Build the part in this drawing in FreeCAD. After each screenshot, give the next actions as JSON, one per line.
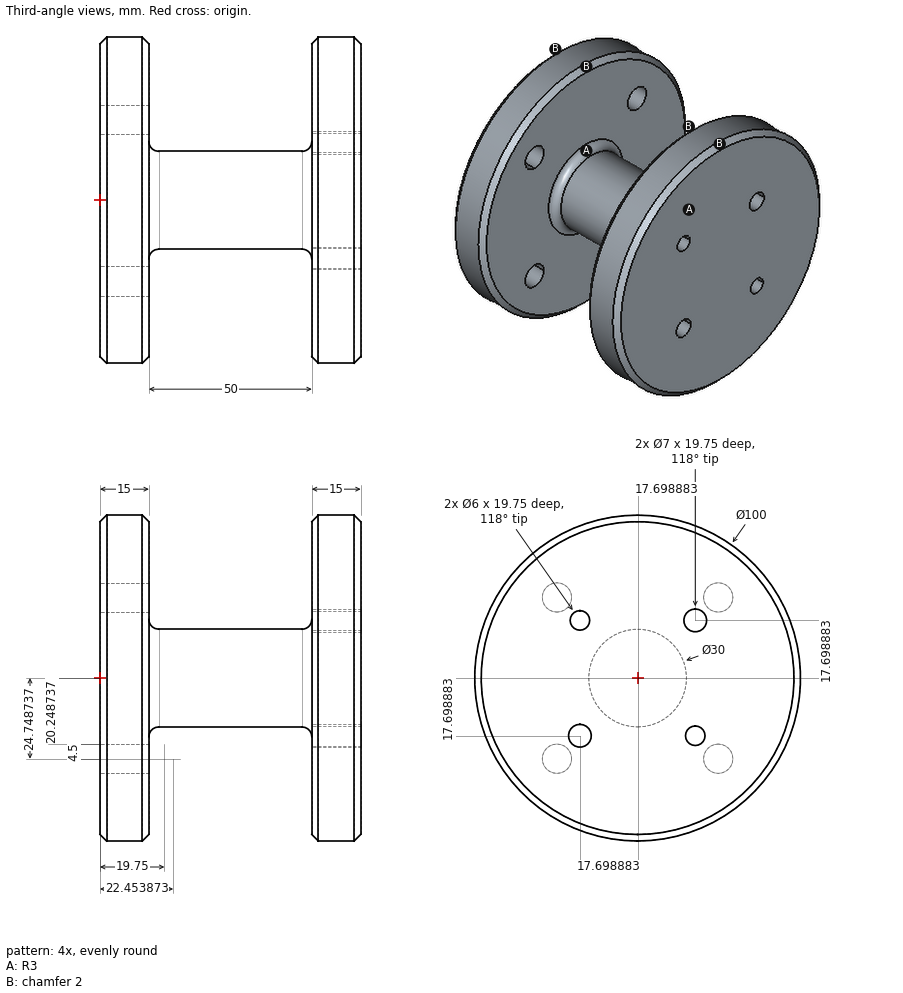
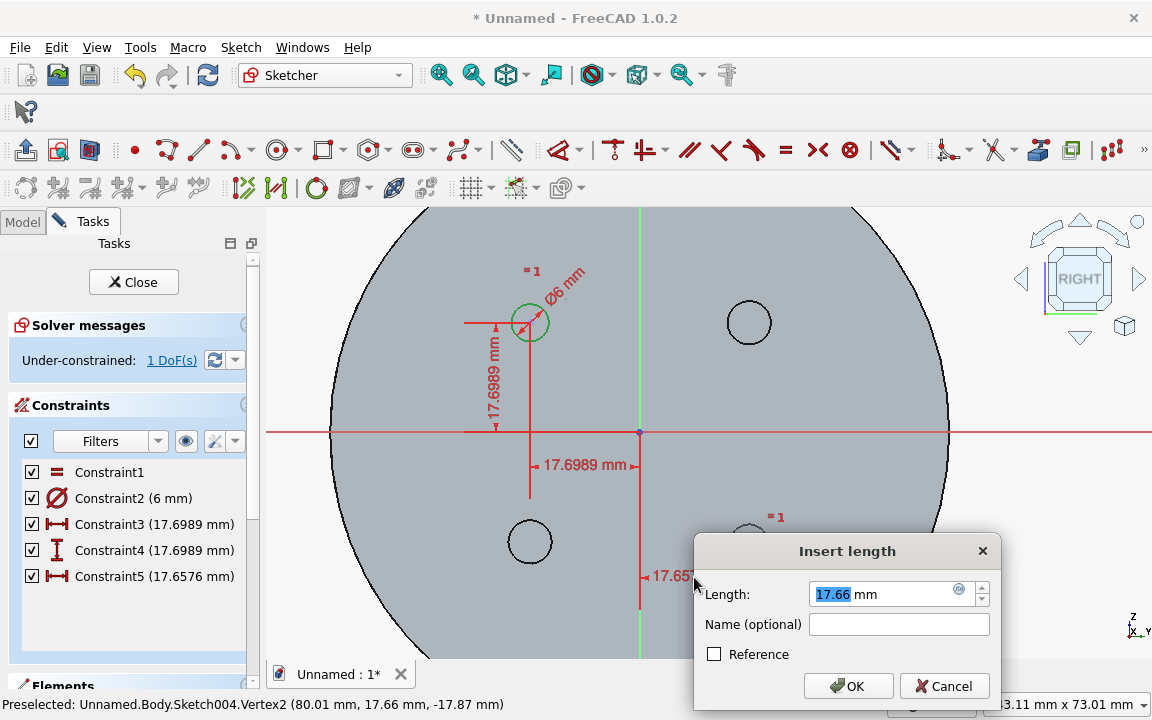
{"action": "type", "text": "17.698883"}
{"action": "key", "text": "Return"}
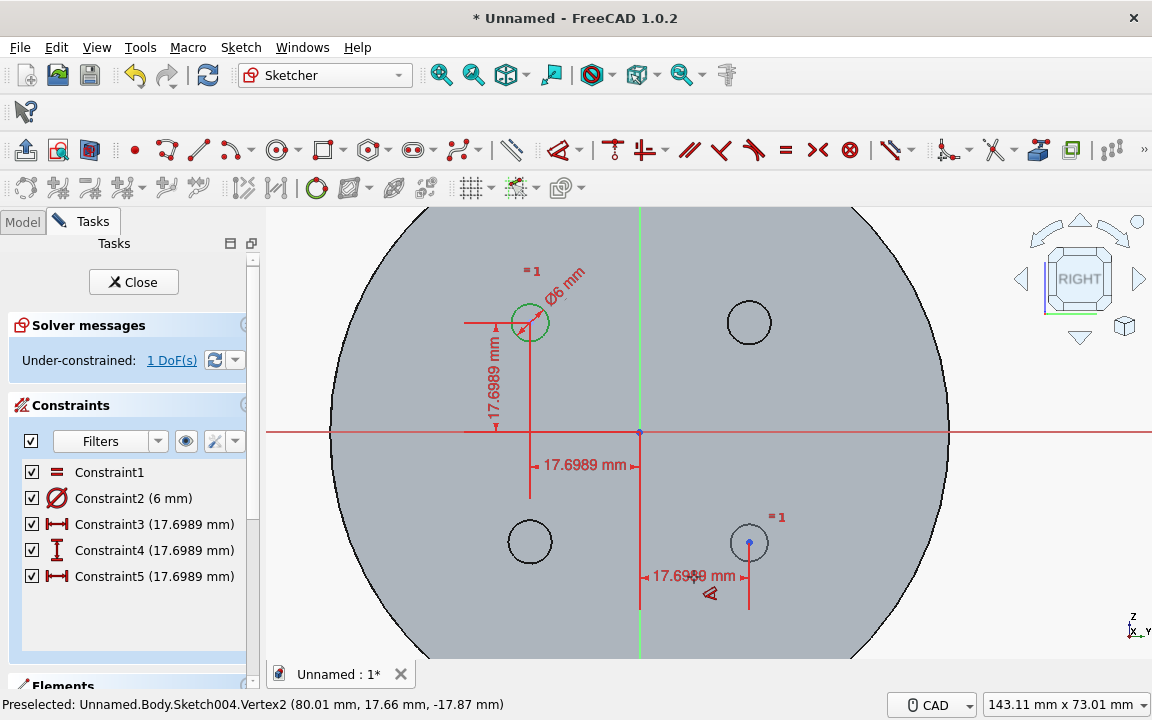
{"action": "left_click", "coordinate": [749, 543]}
{"action": "left_click", "coordinate": [783, 488]}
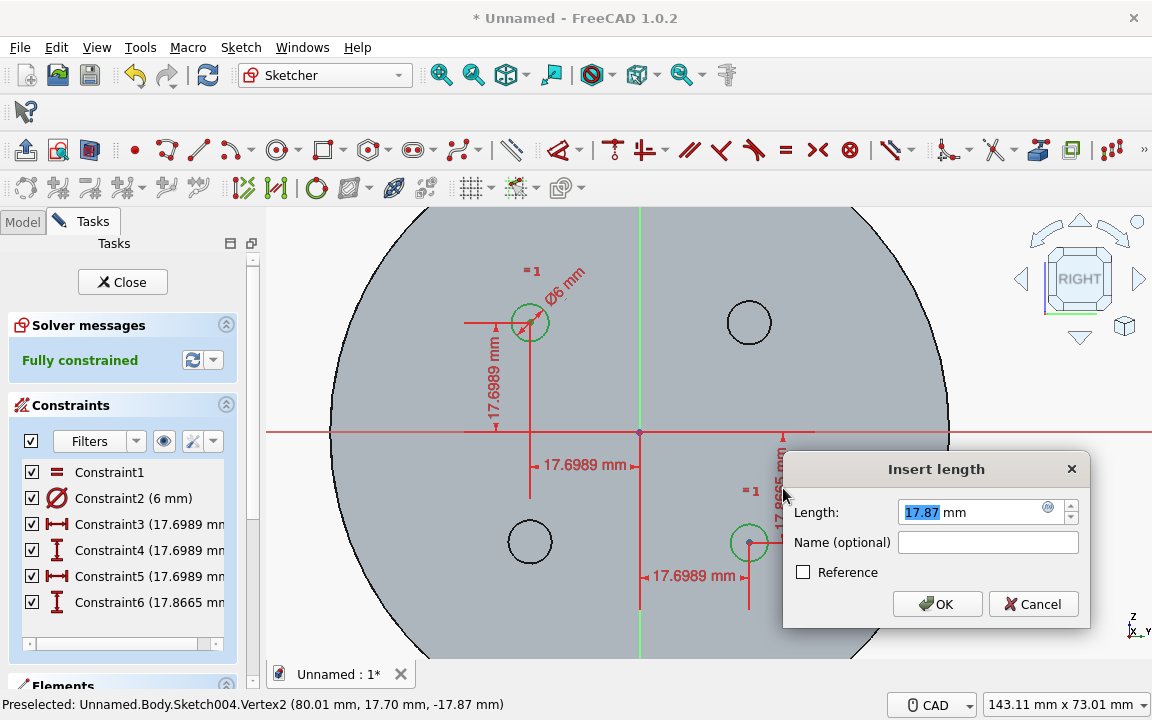
{"action": "type", "text": "17.698883"}
{"action": "key", "text": "Return"}
{"action": "key", "text": "Escape"}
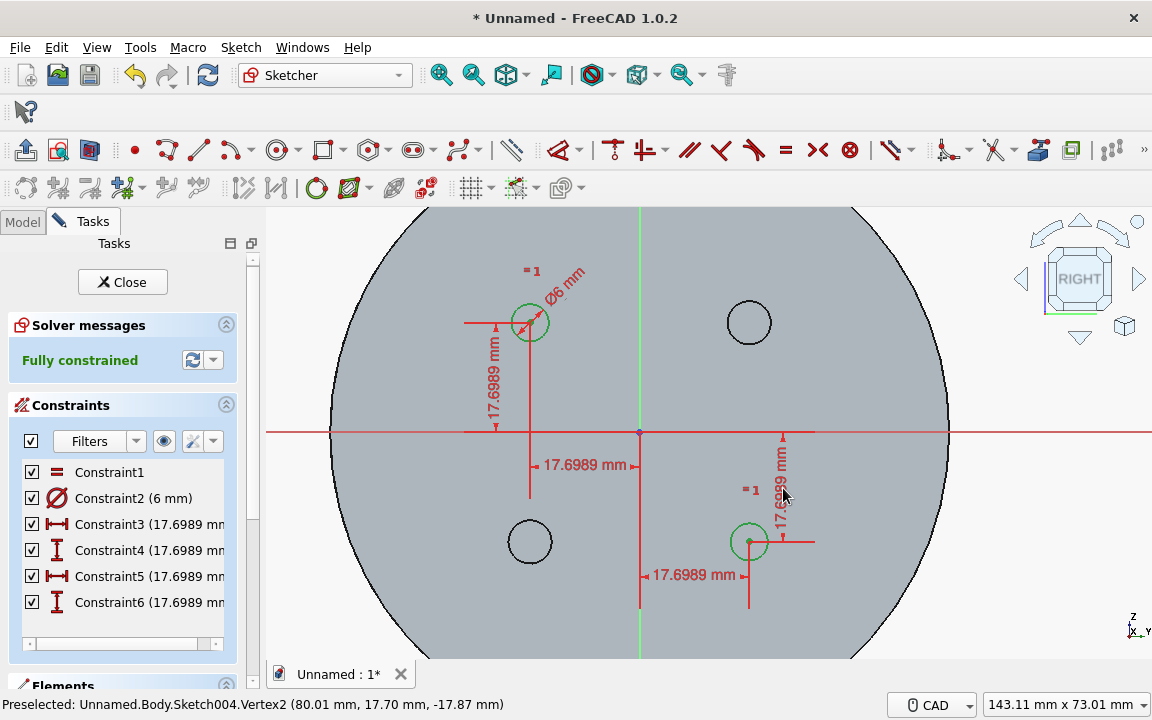
{"action": "left_click", "coordinate": [123, 282]}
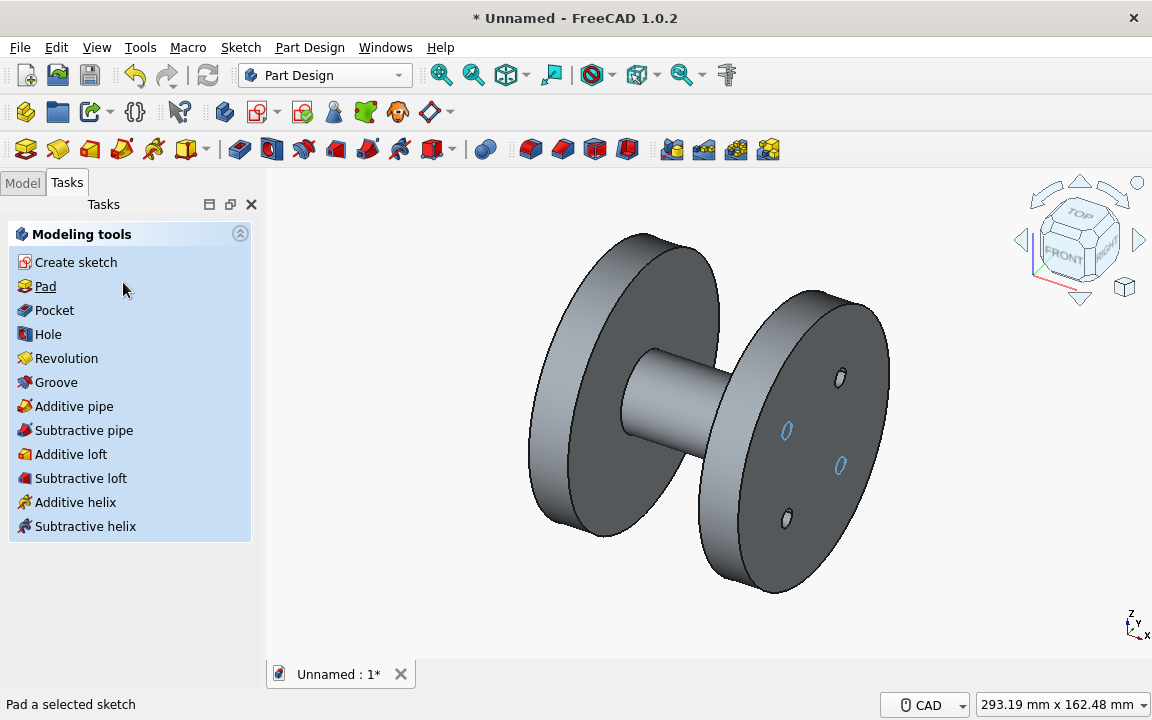
{"action": "left_click", "coordinate": [272, 150]}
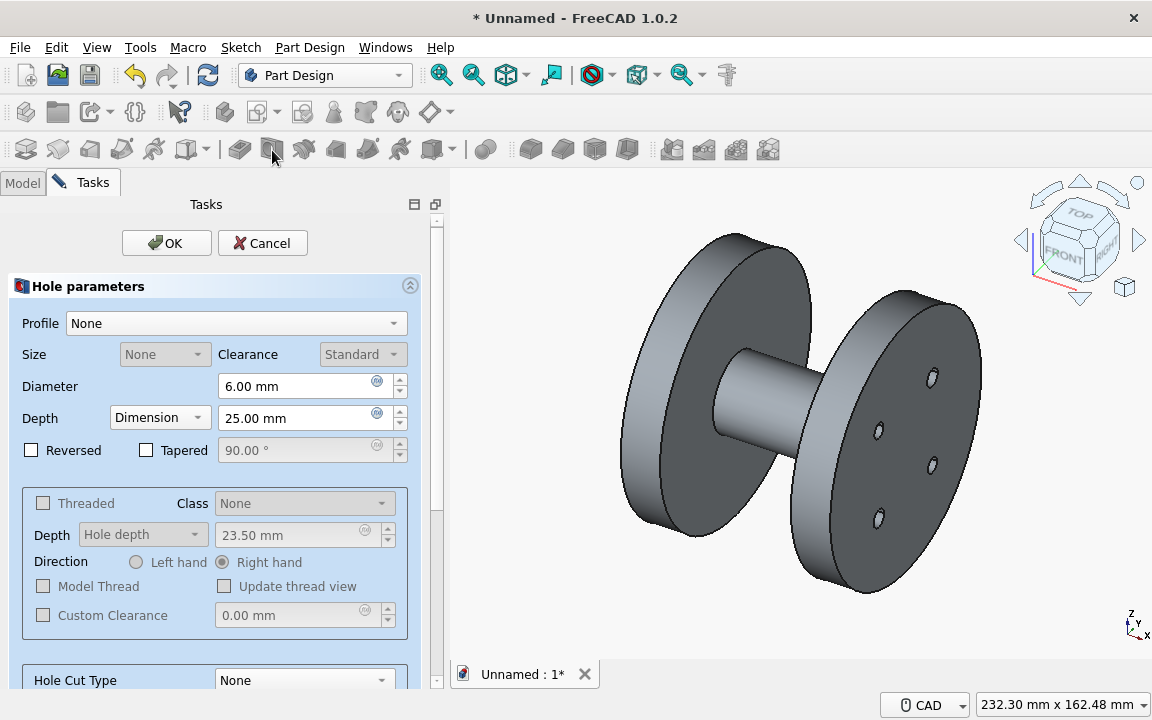
{"action": "triple_click", "coordinate": [305, 386]}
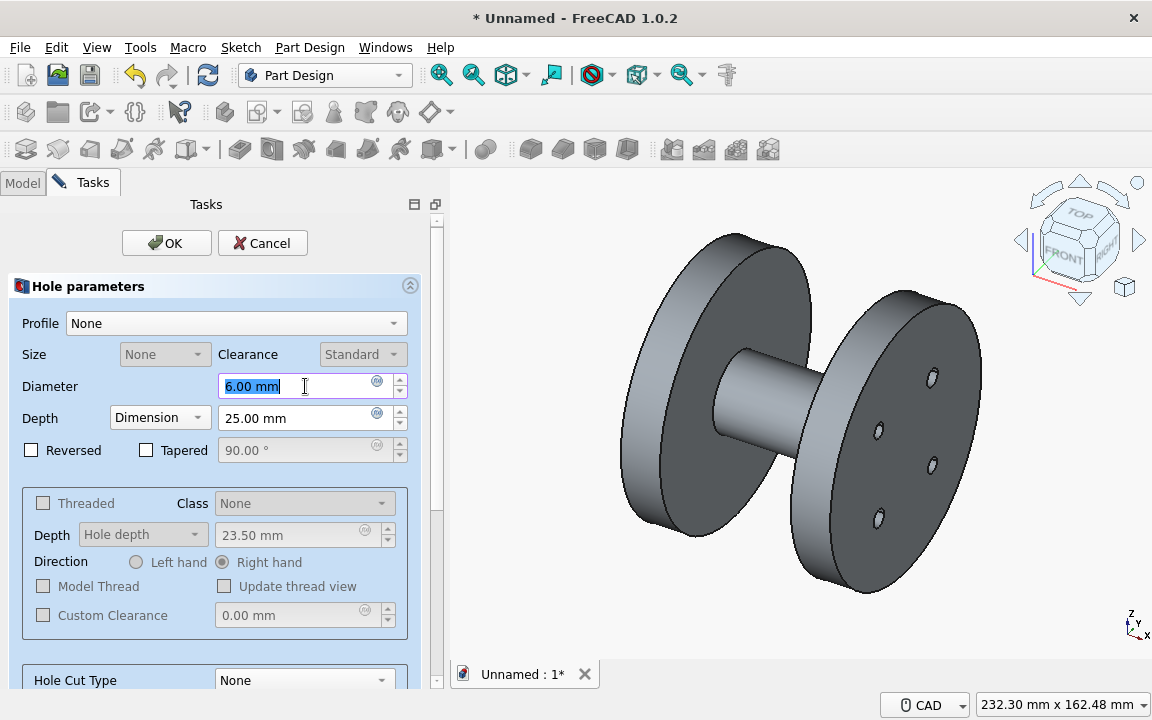
{"action": "type", "text": "6"}
{"action": "key", "text": "Tab"}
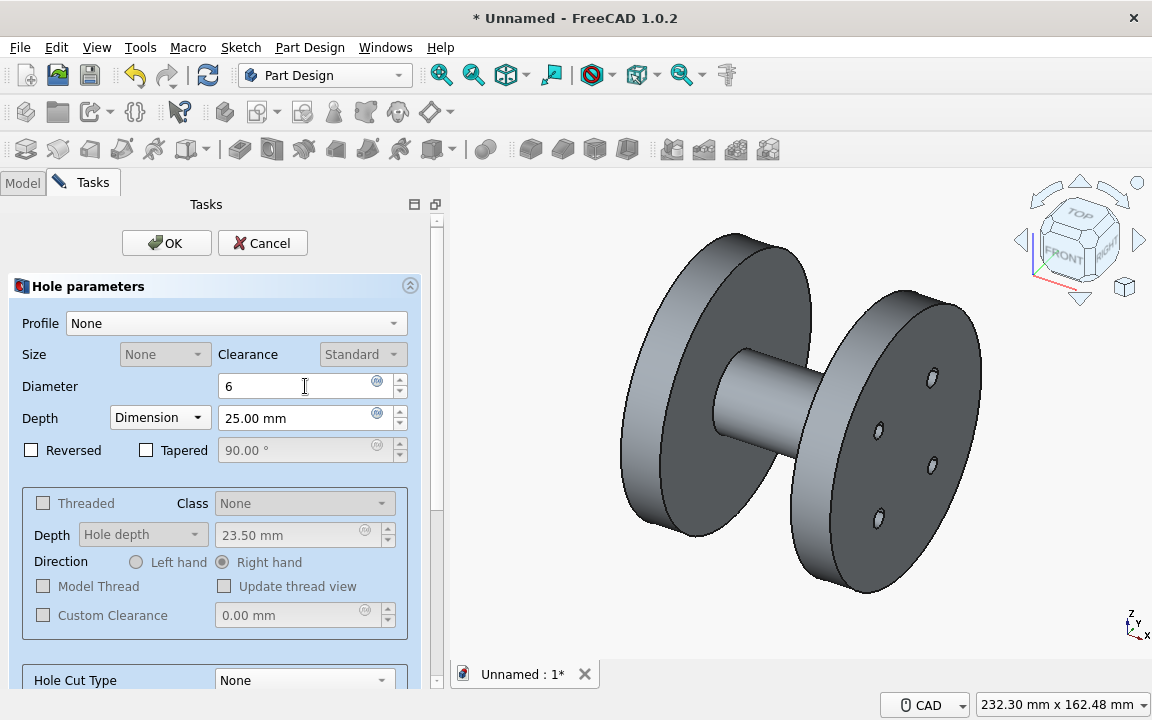
{"action": "triple_click", "coordinate": [305, 418]}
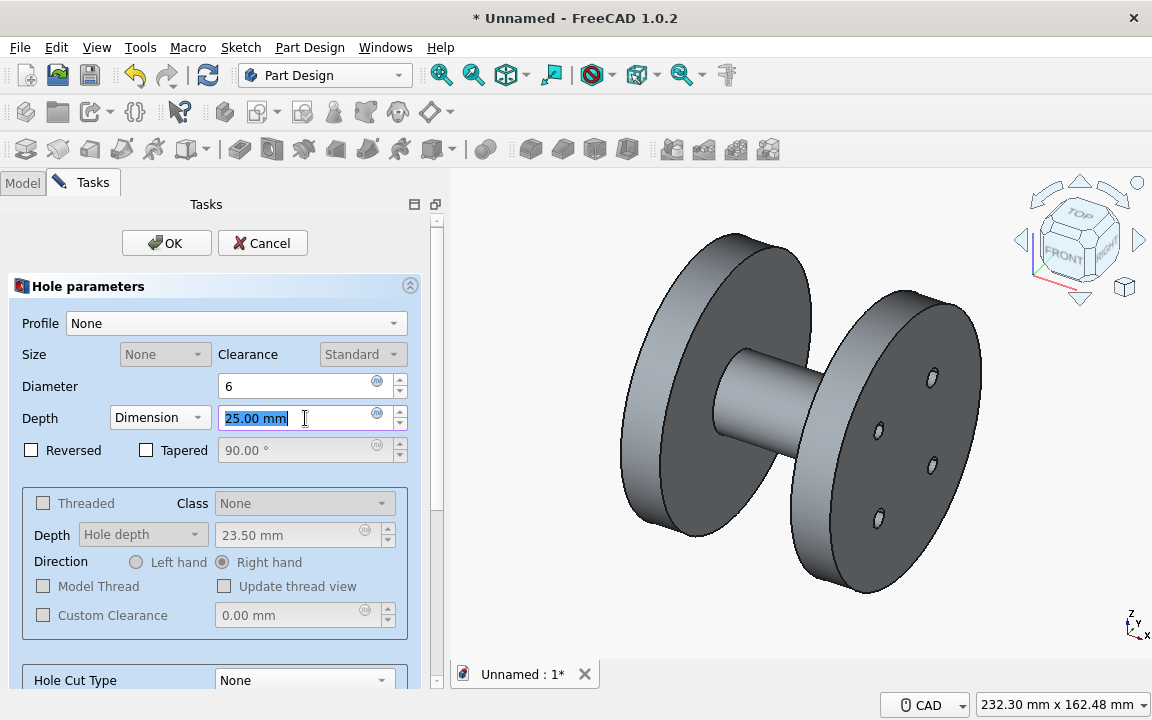
{"action": "type", "text": "19.75"}
{"action": "key", "text": "Tab"}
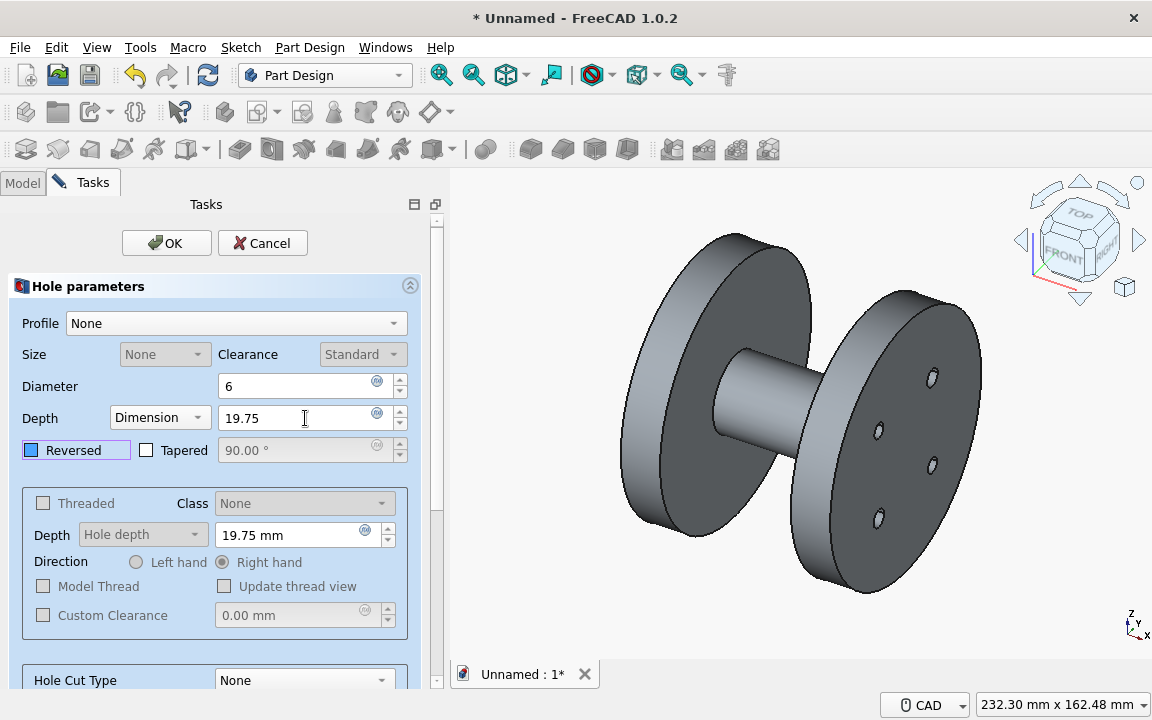
{"action": "left_click", "coordinate": [167, 243]}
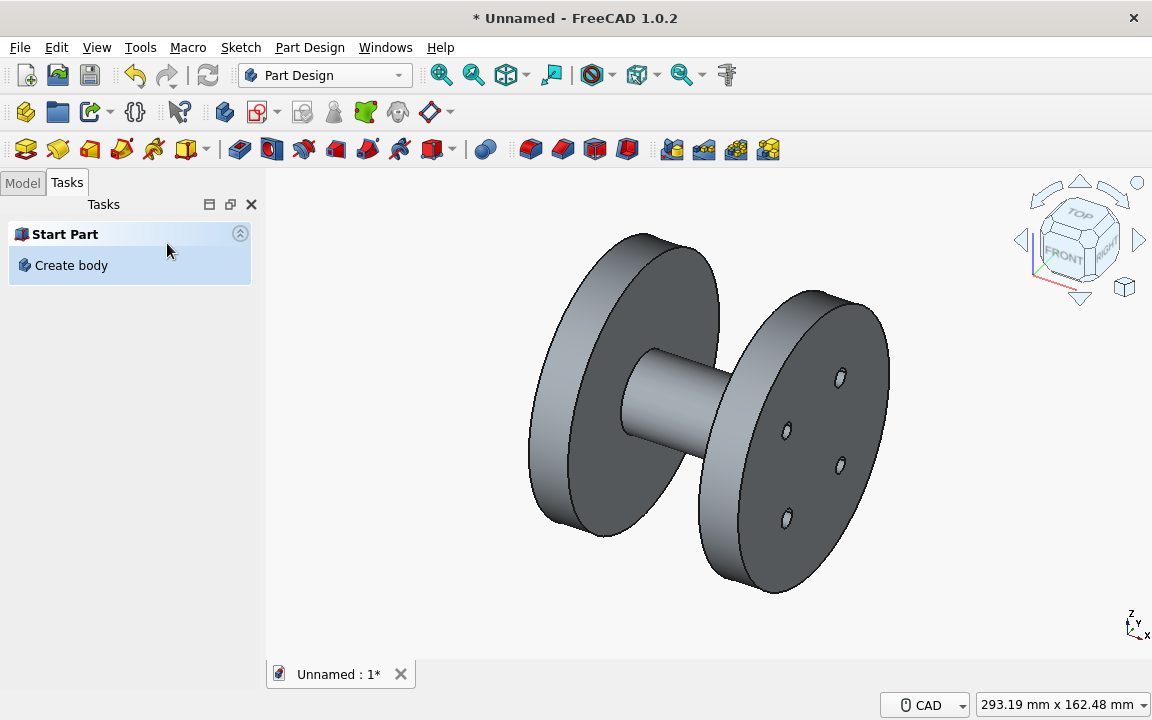
{"action": "left_click", "coordinate": [23, 182]}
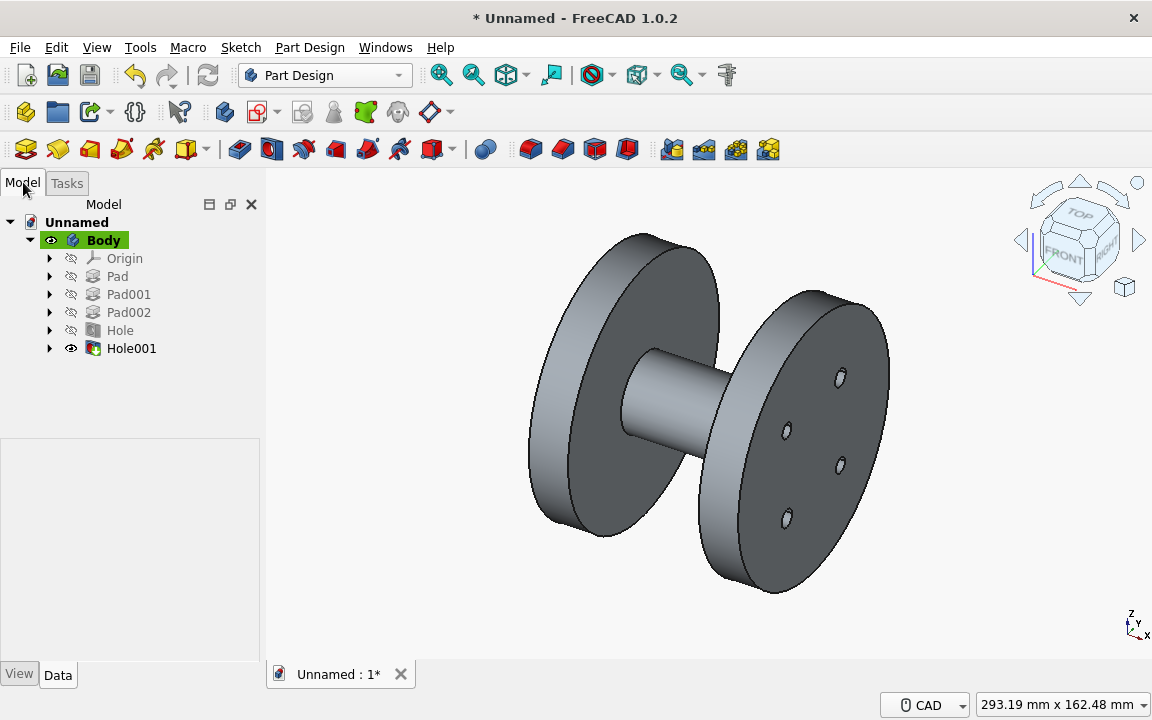
{"action": "left_click", "coordinate": [50, 258]}